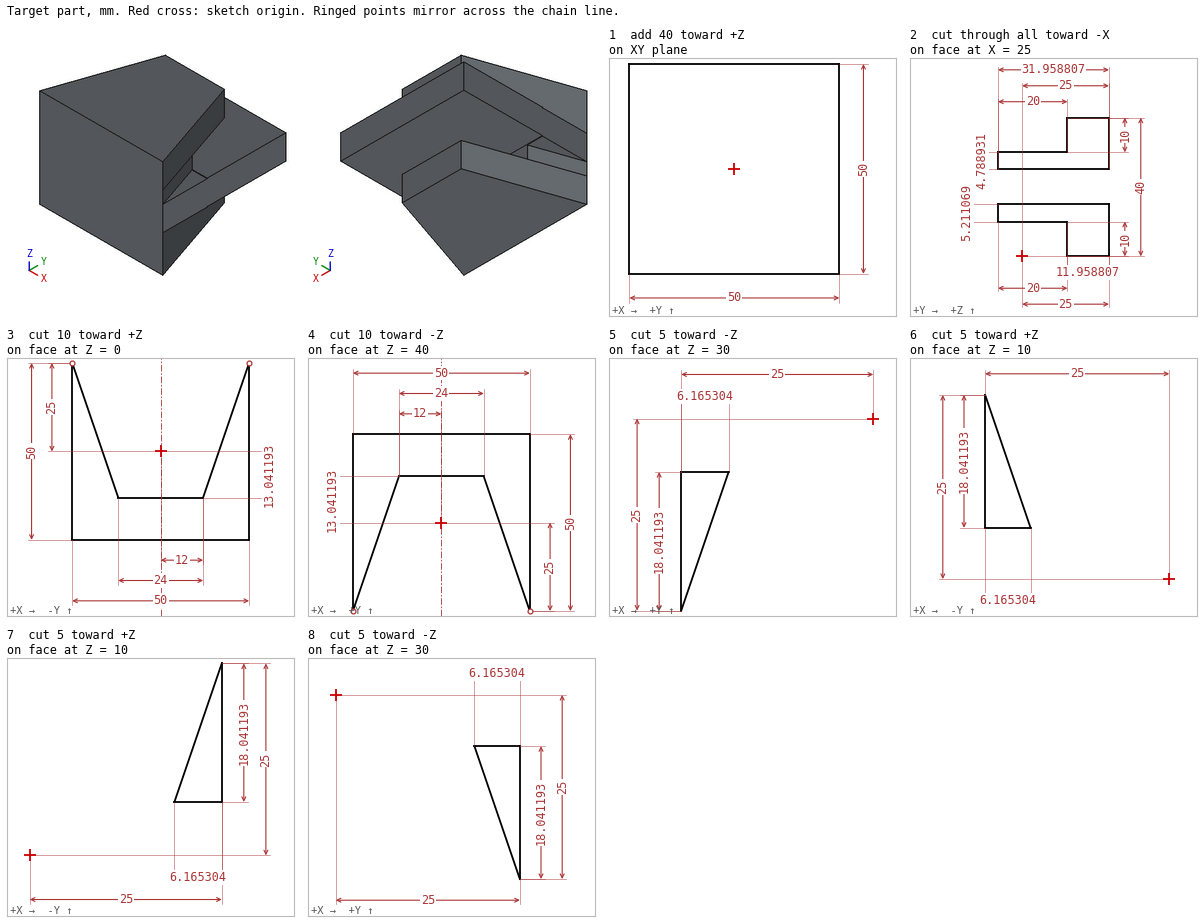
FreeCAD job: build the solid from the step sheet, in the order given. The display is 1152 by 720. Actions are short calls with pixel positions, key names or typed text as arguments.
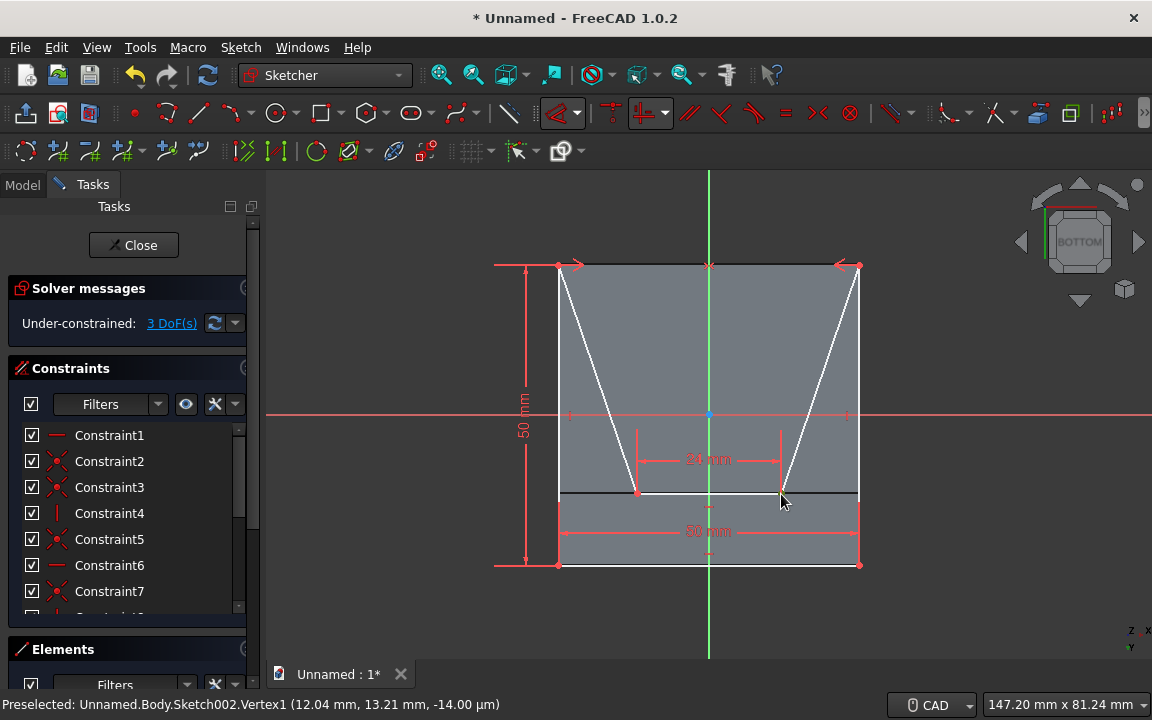
key(l)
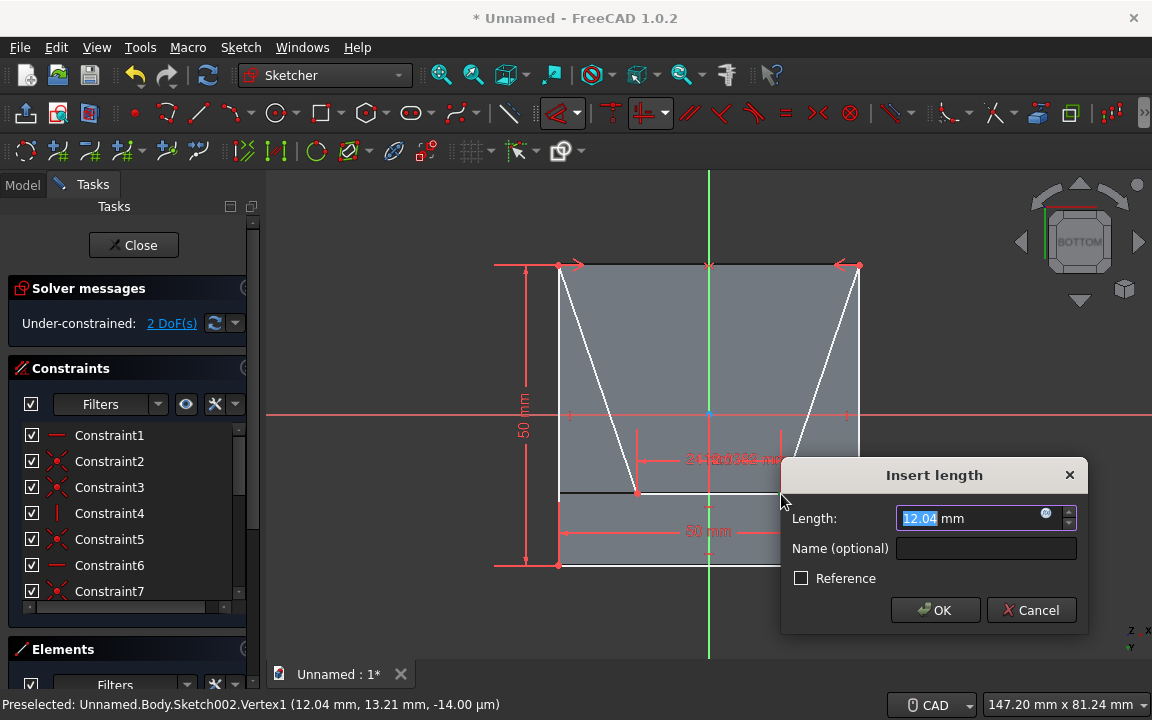
text(12)
key(Return)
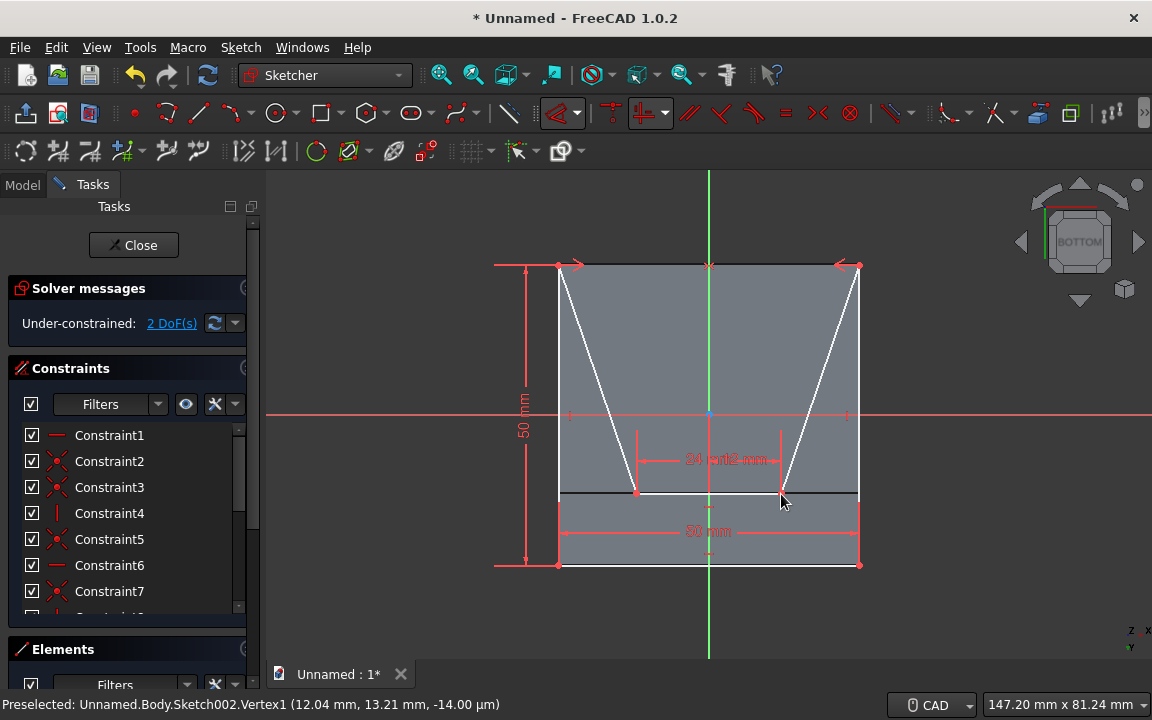
click(559, 265)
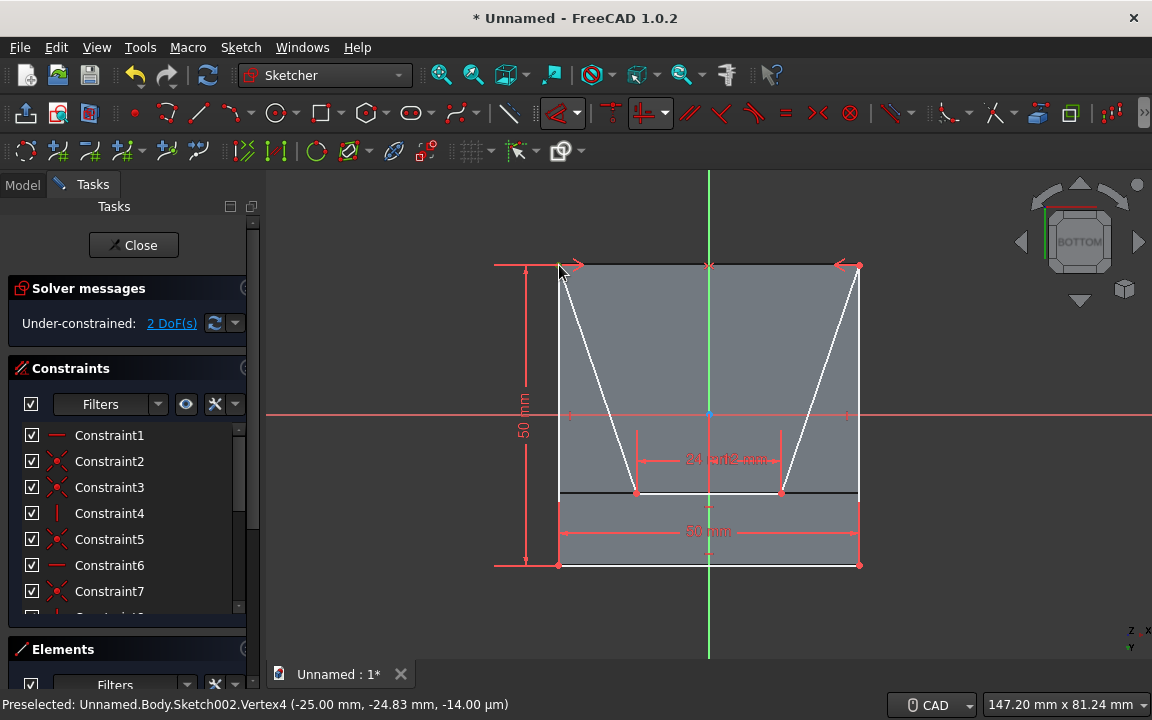
key(i)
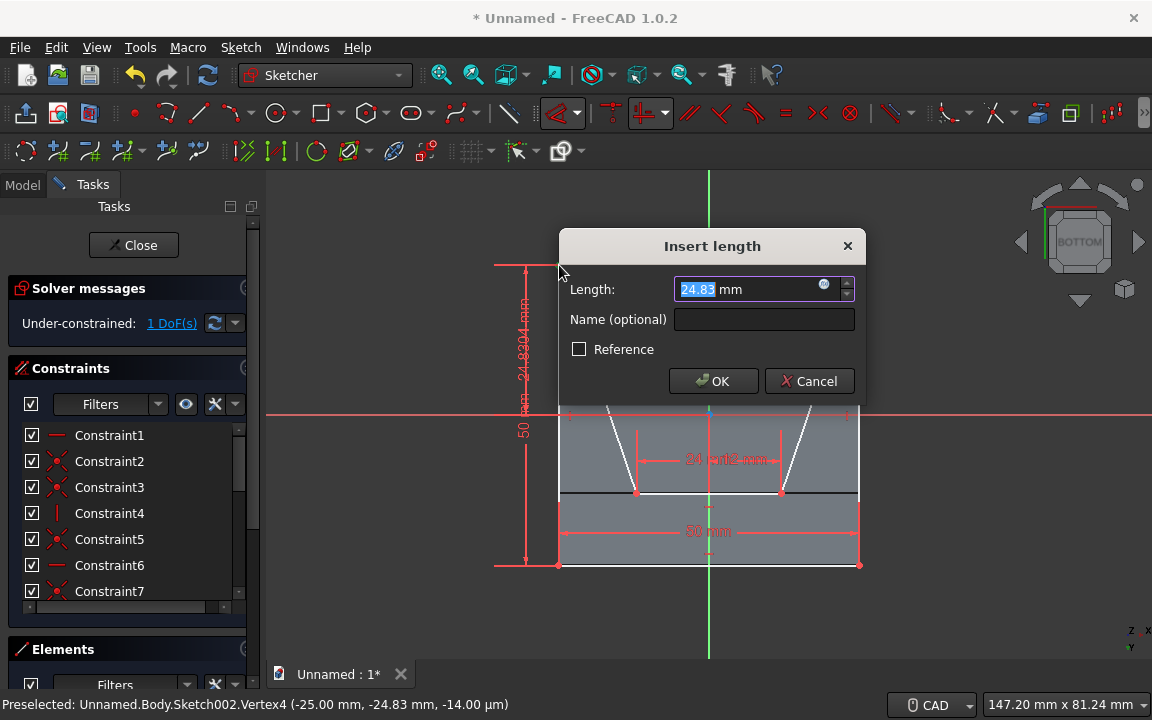
text(25)
key(Return)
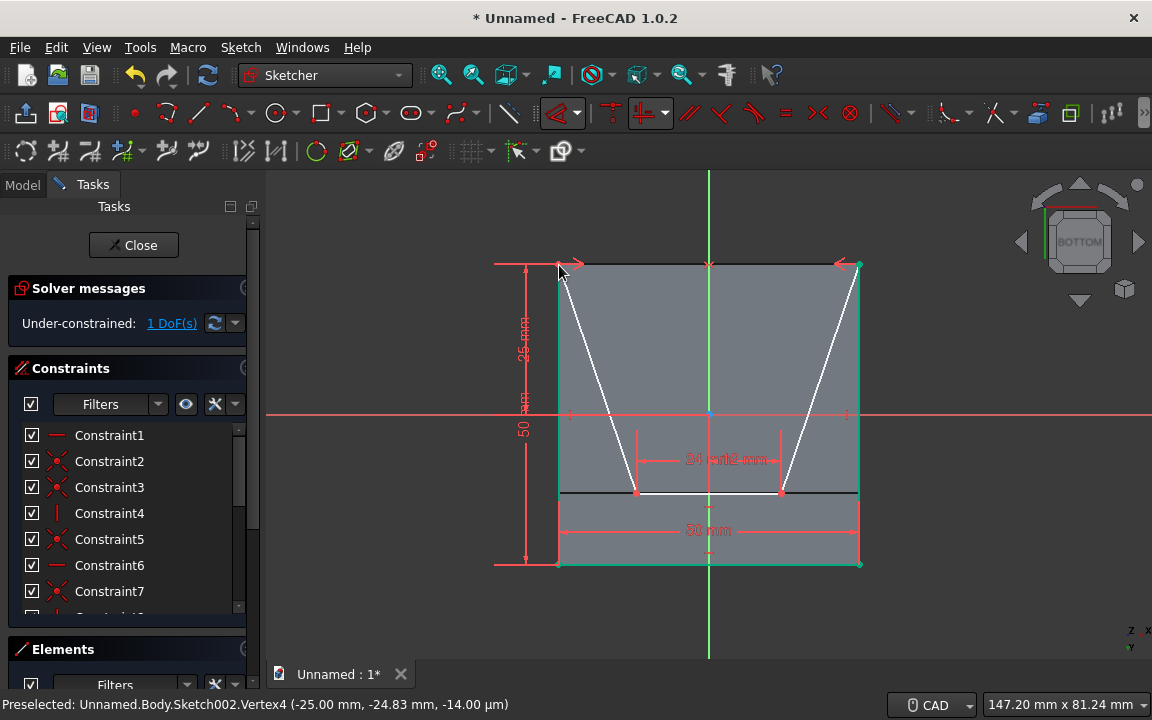
click(781, 494)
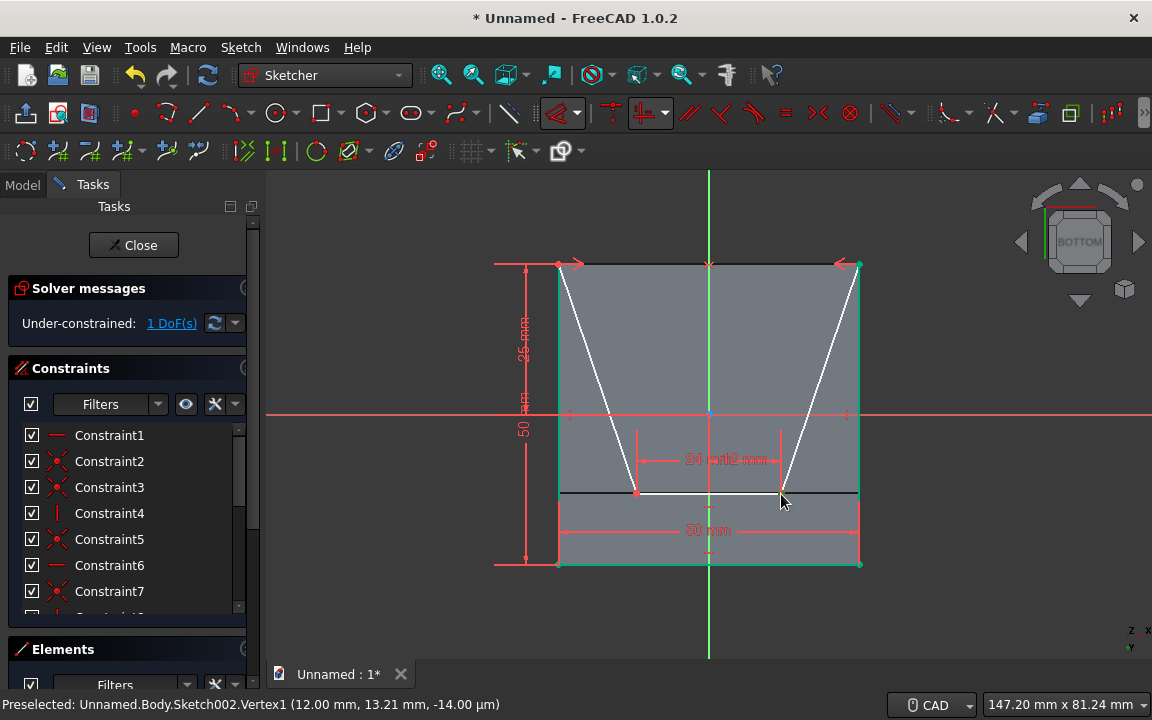
key(i)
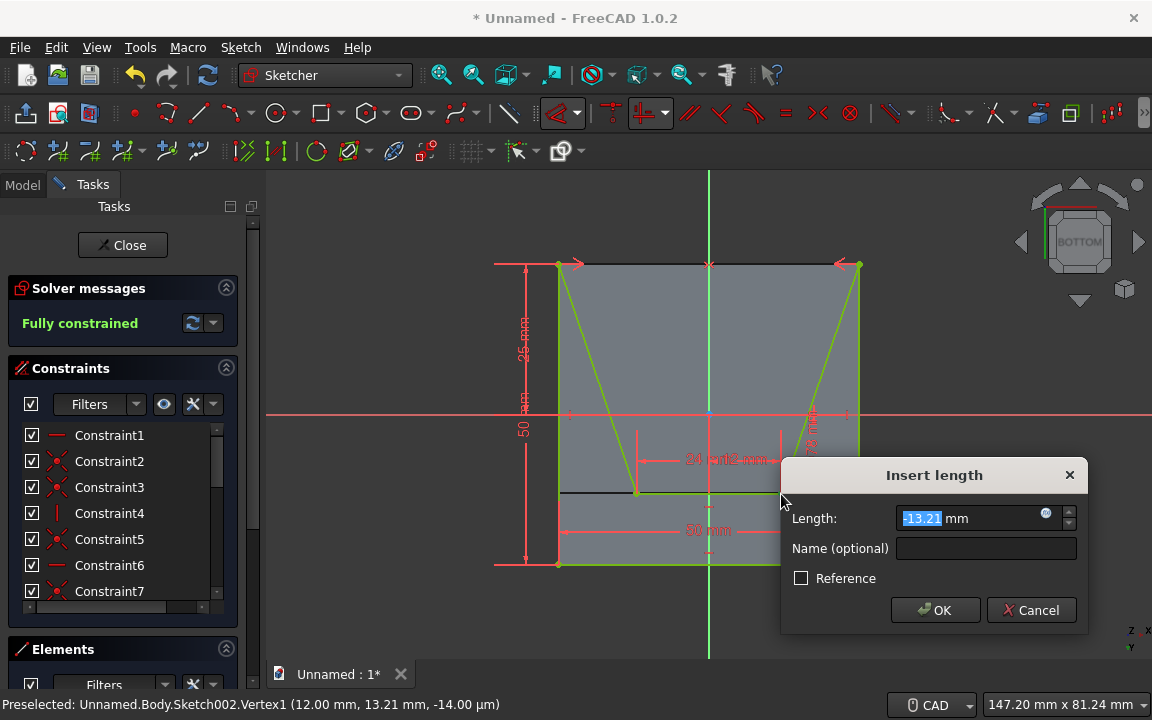
text(-13.041193)
key(Return)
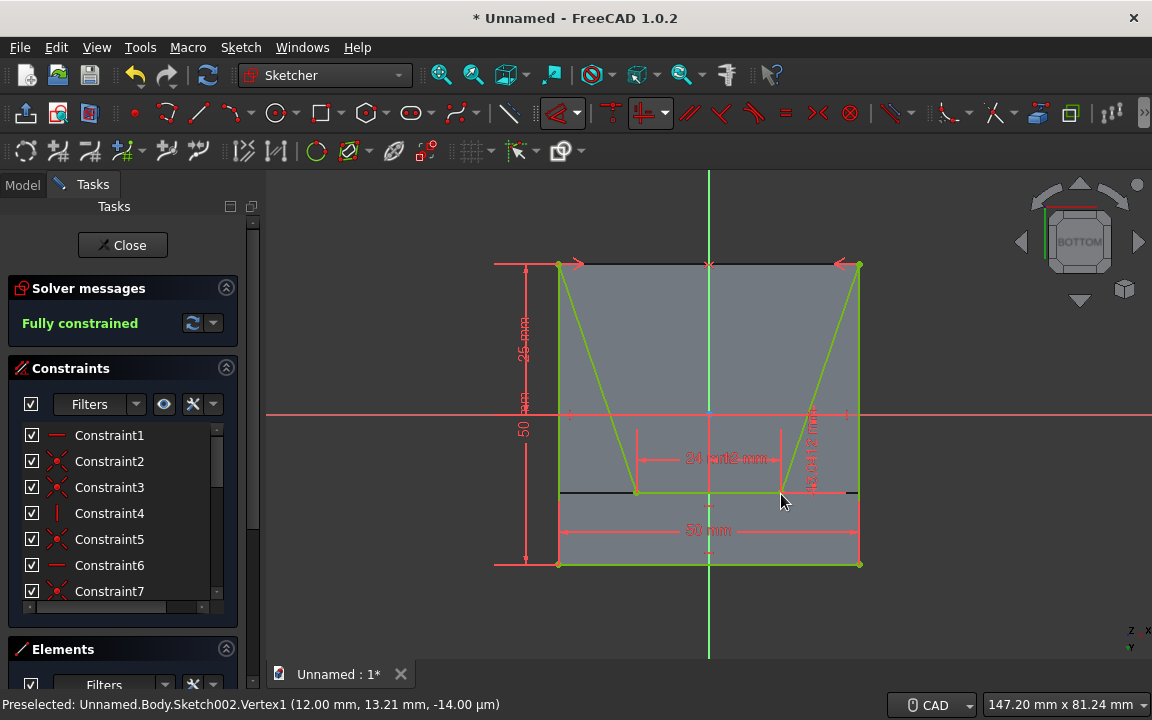
click(123, 245)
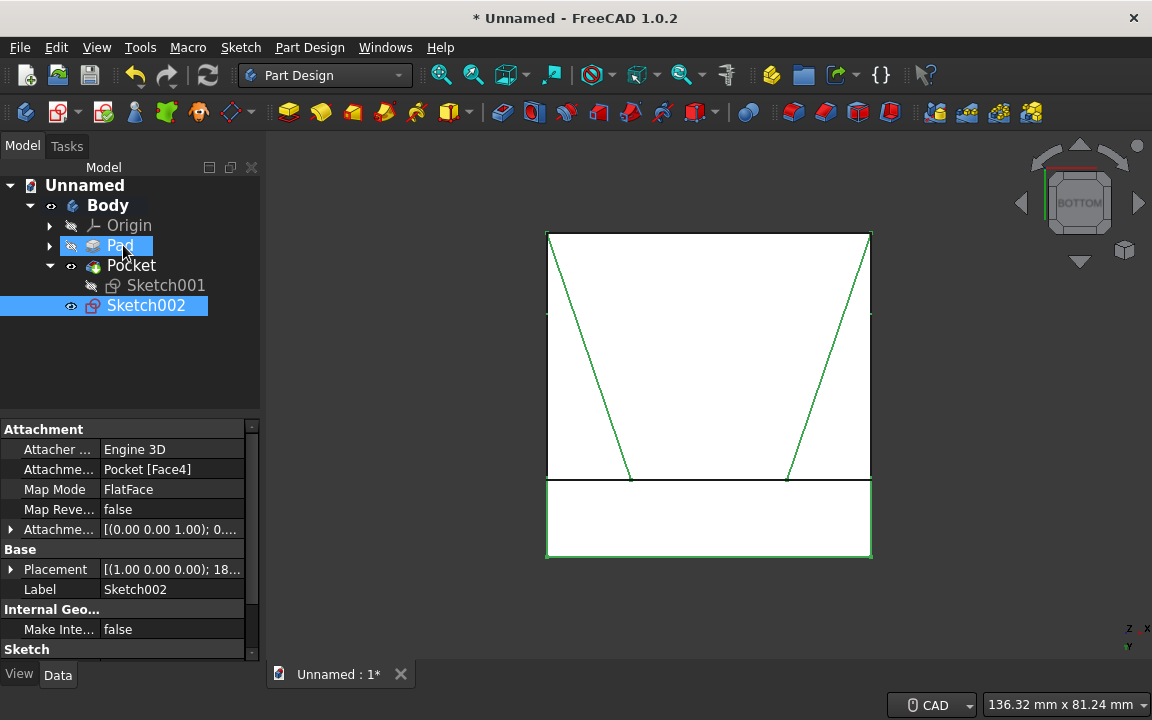
click(504, 112)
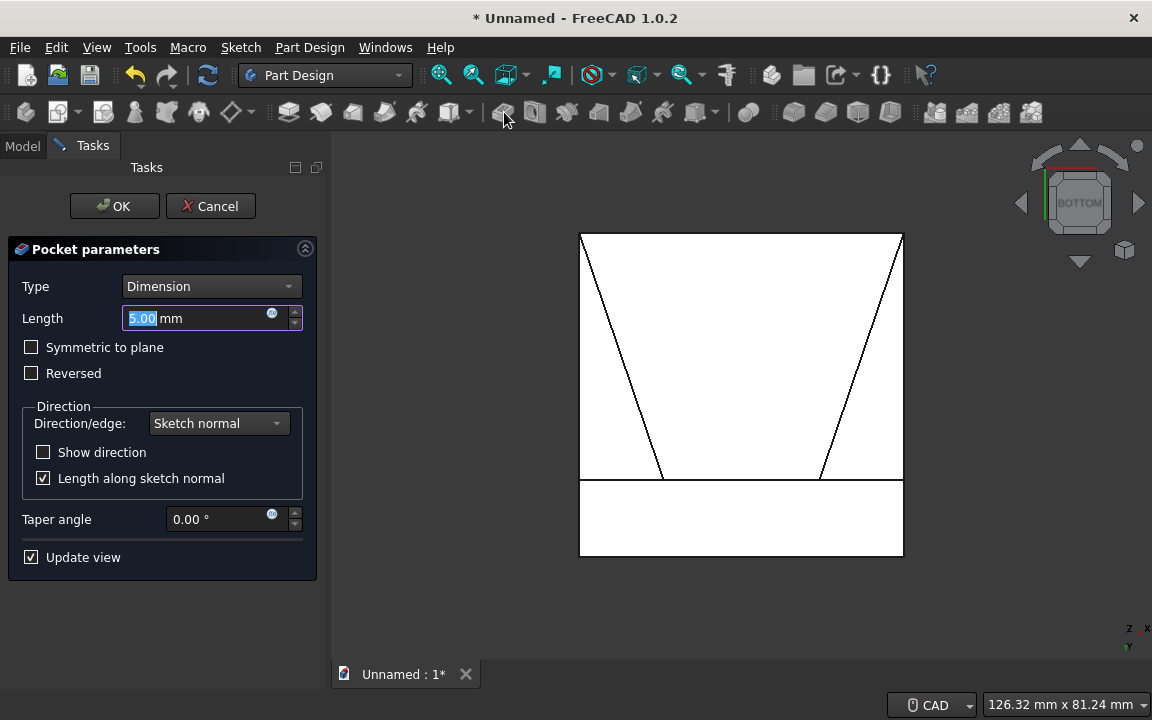
text(10)
key(Tab)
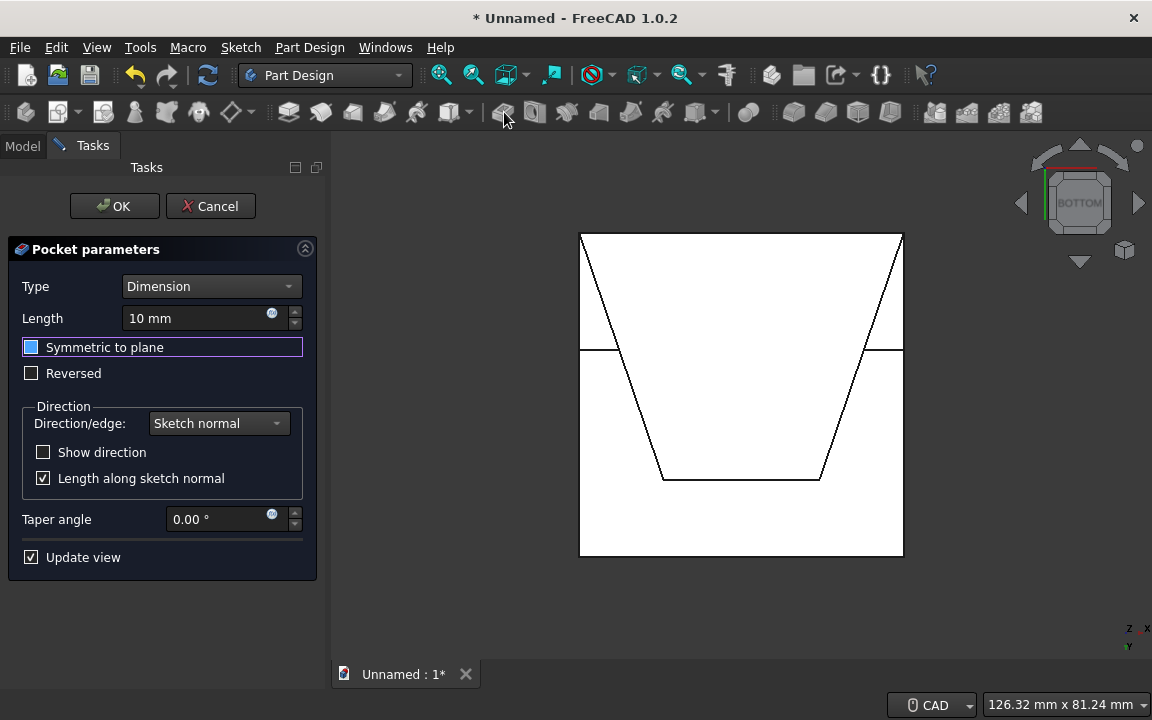
click(115, 206)